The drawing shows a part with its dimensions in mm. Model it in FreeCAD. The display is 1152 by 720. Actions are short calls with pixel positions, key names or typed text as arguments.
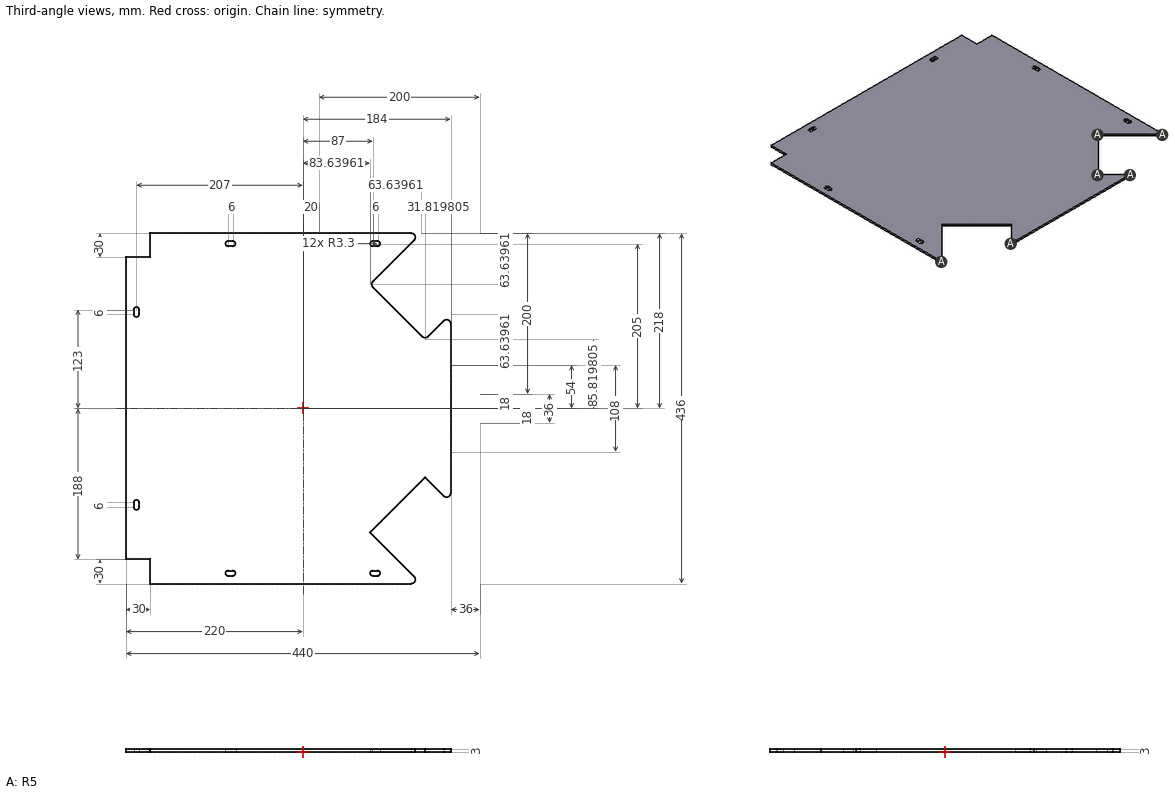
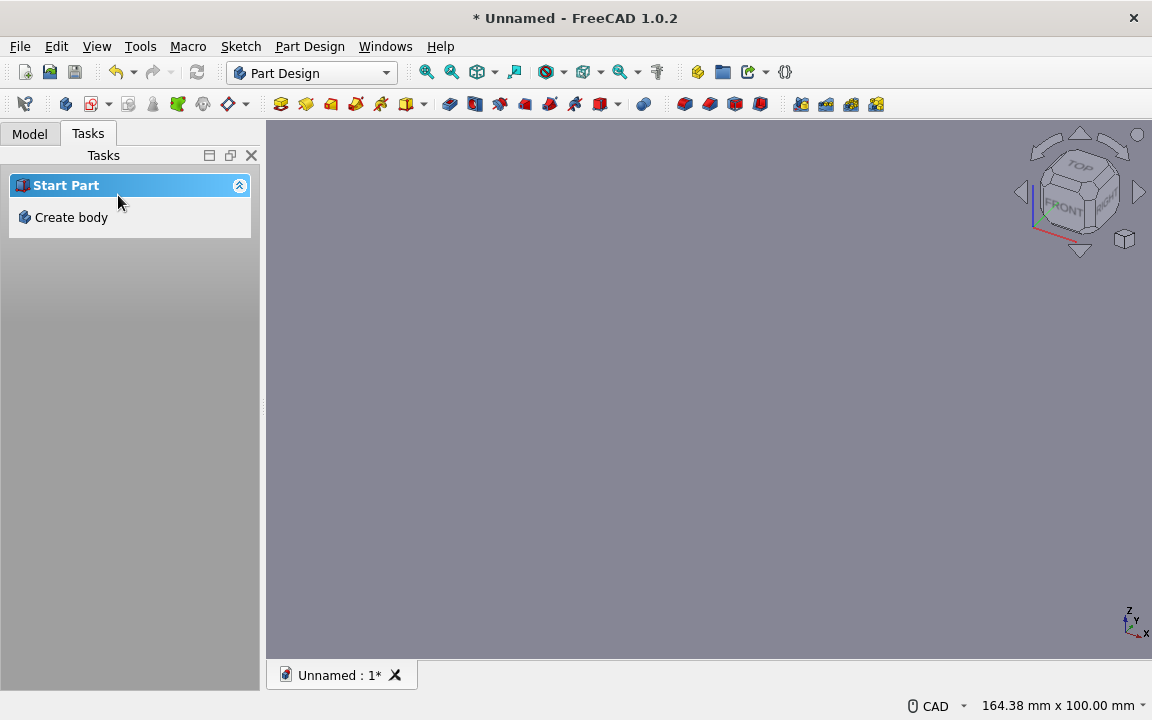
key(v)
key(f)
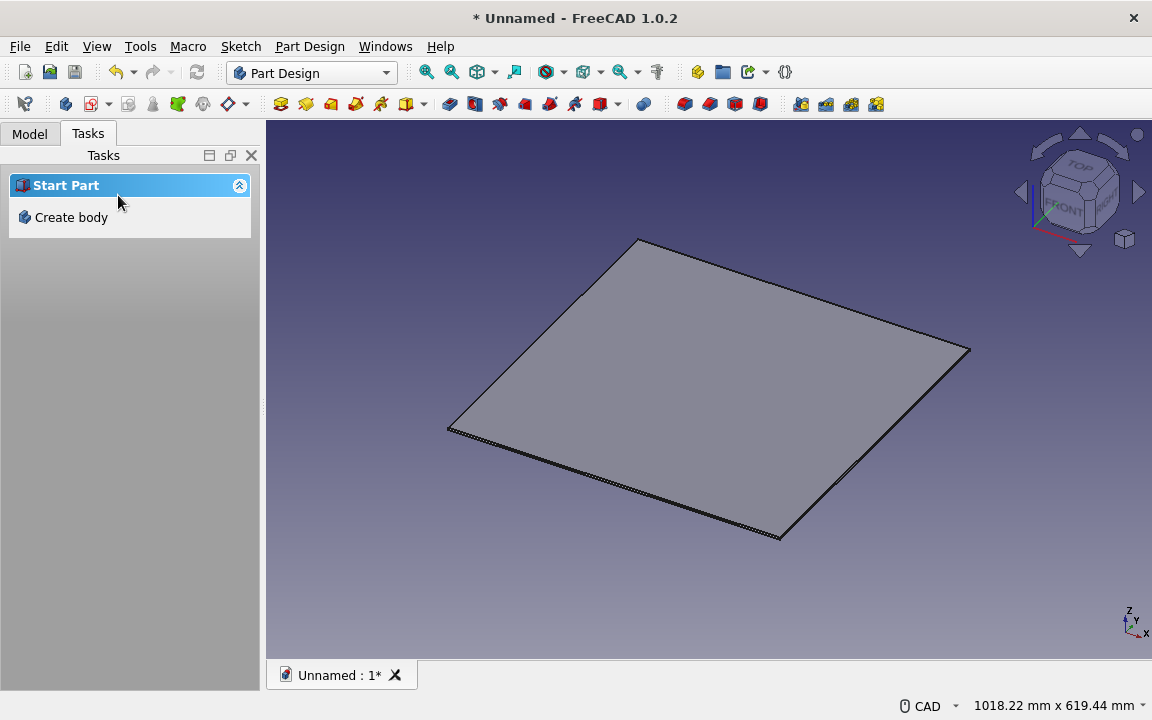
click(709, 387)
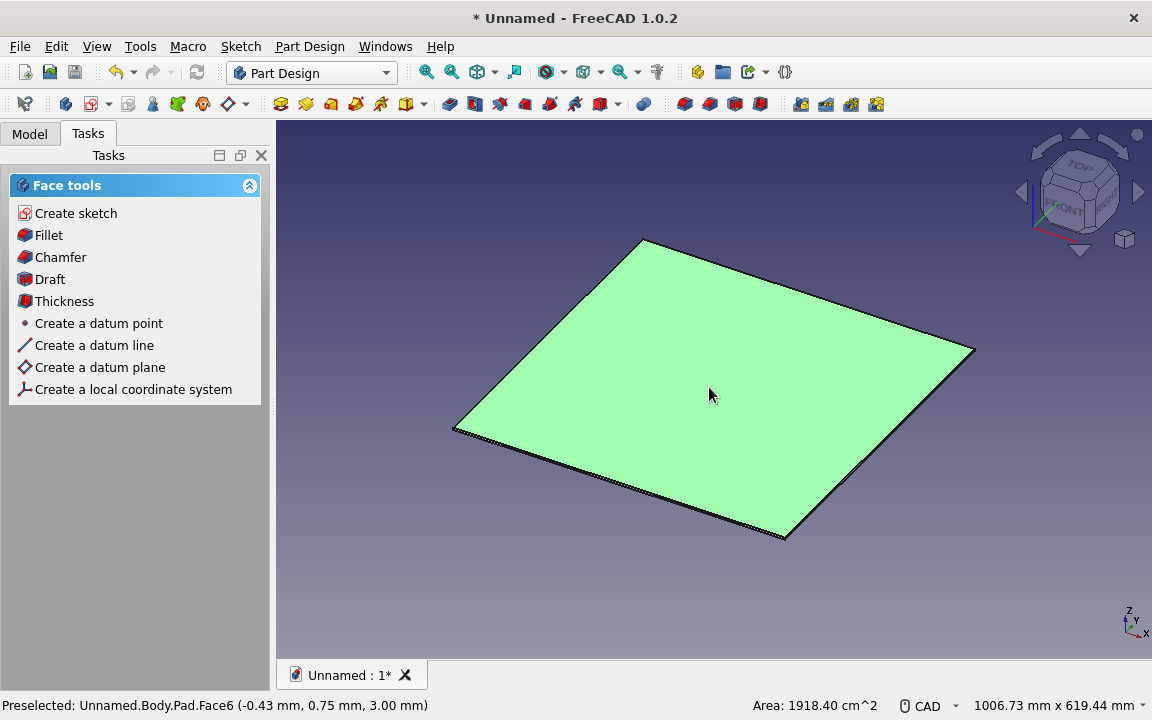
click(90, 104)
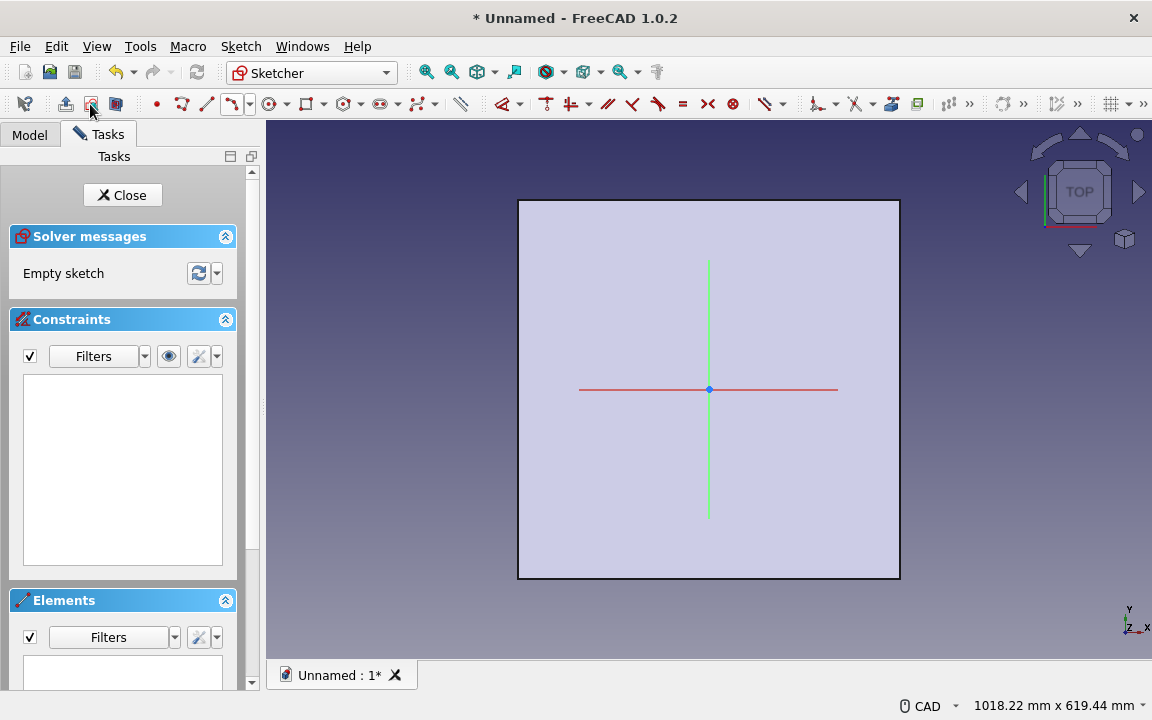
key(g)
key(r)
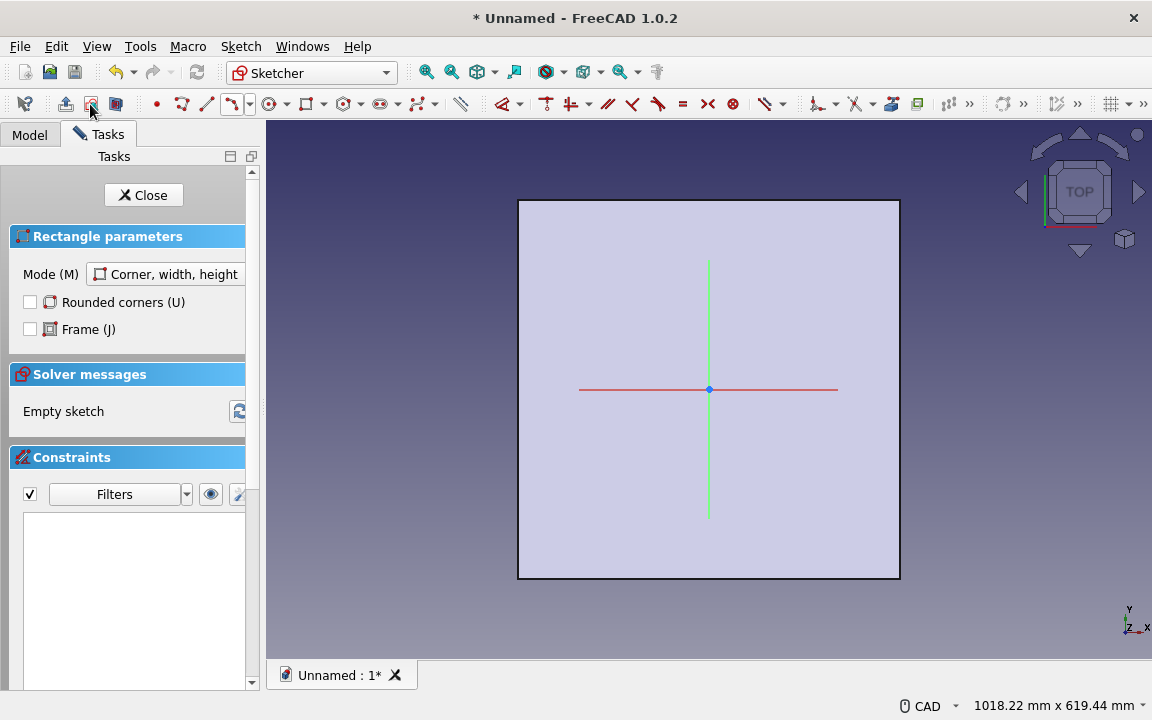
click(518, 553)
move(544, 579)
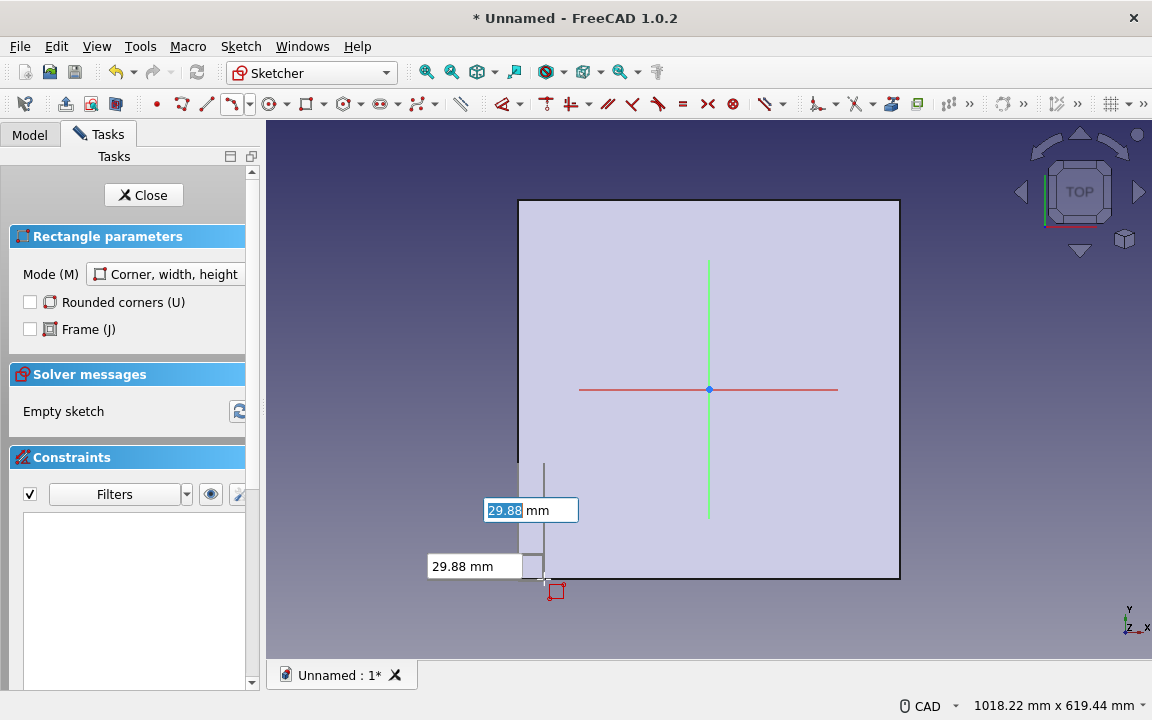
text(30)
key(Tab)
text(30)
key(Return)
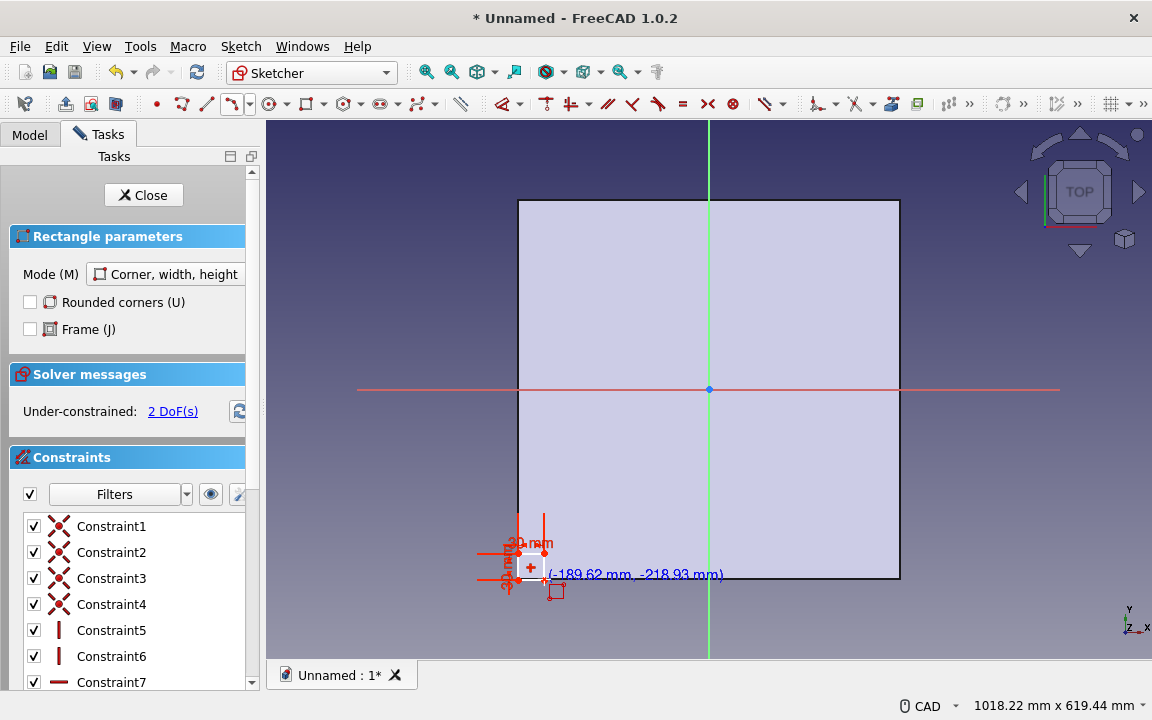
click(518, 200)
move(544, 226)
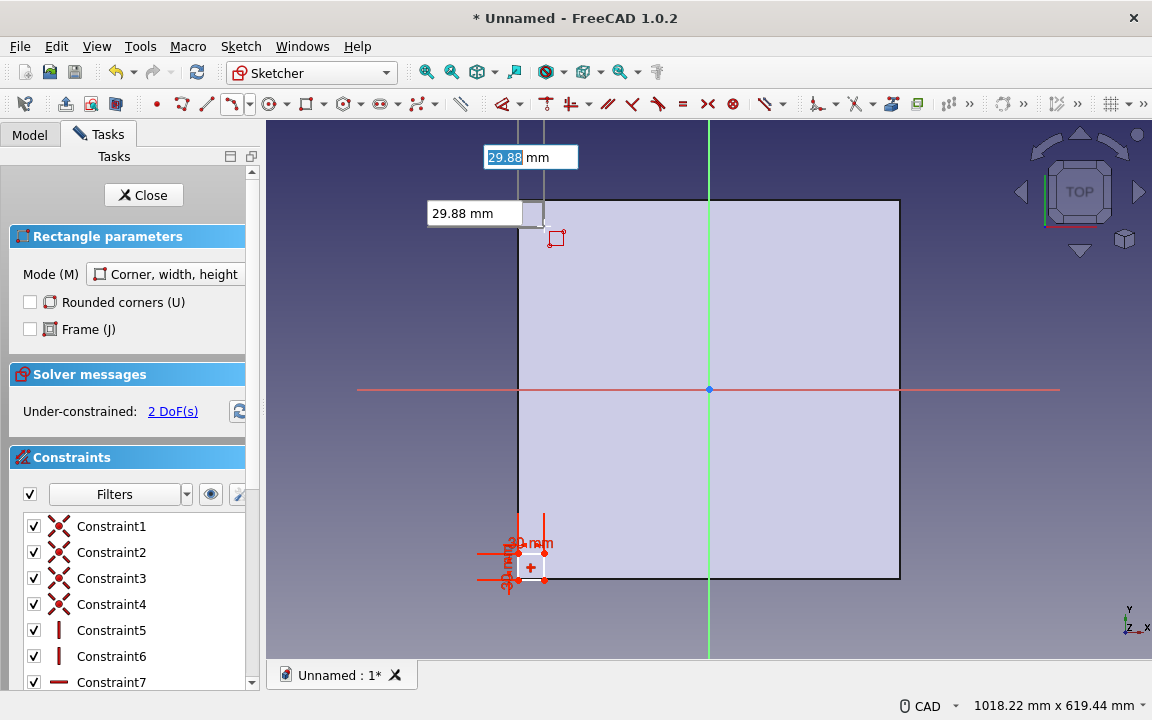
text(30)
key(Tab)
text(30)
key(Return)
key(Escape)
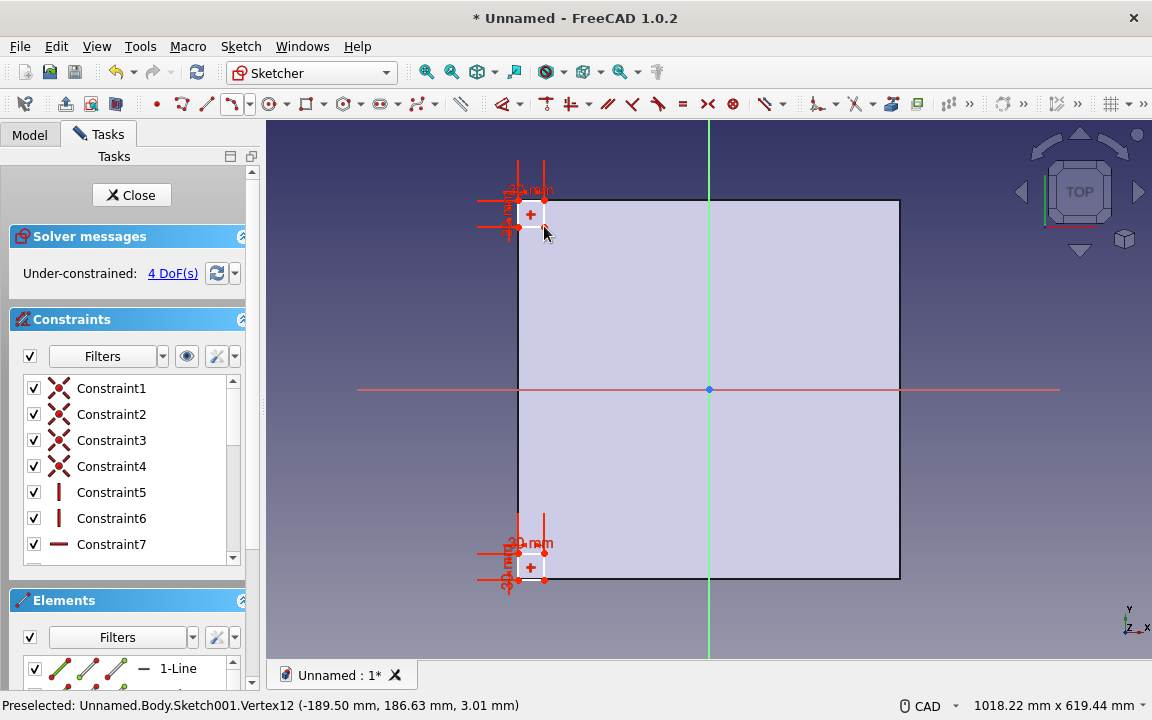
click(518, 580)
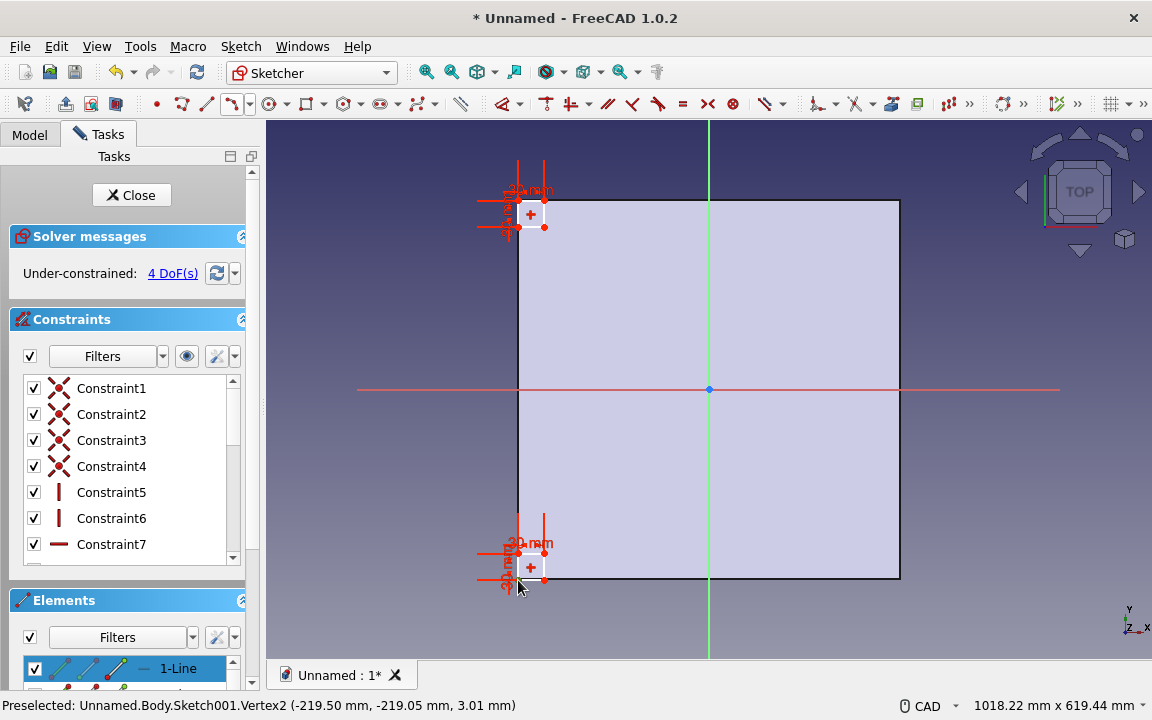
click(518, 201)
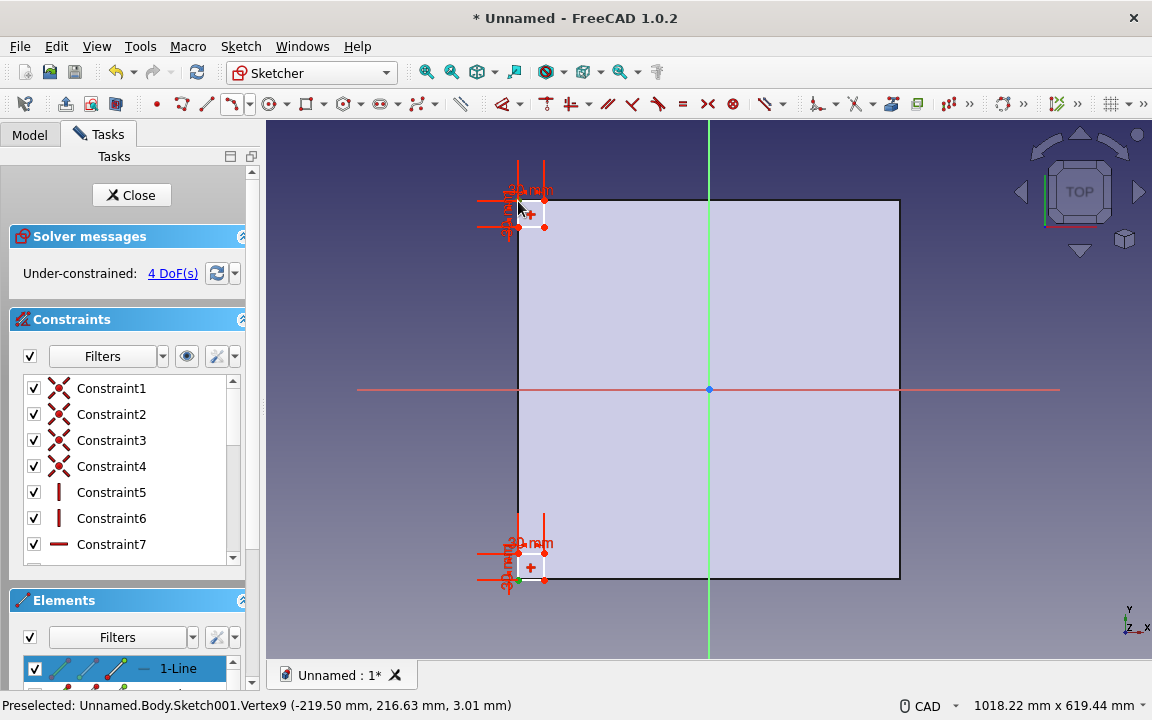
click(393, 390)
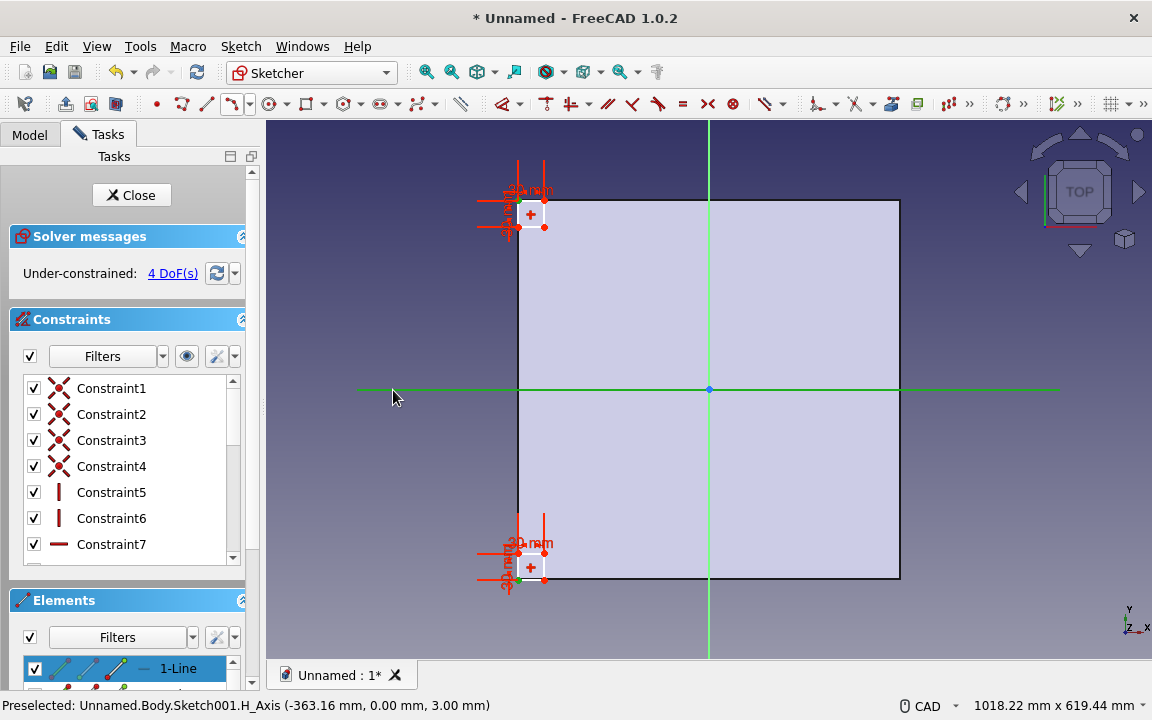
click(708, 104)